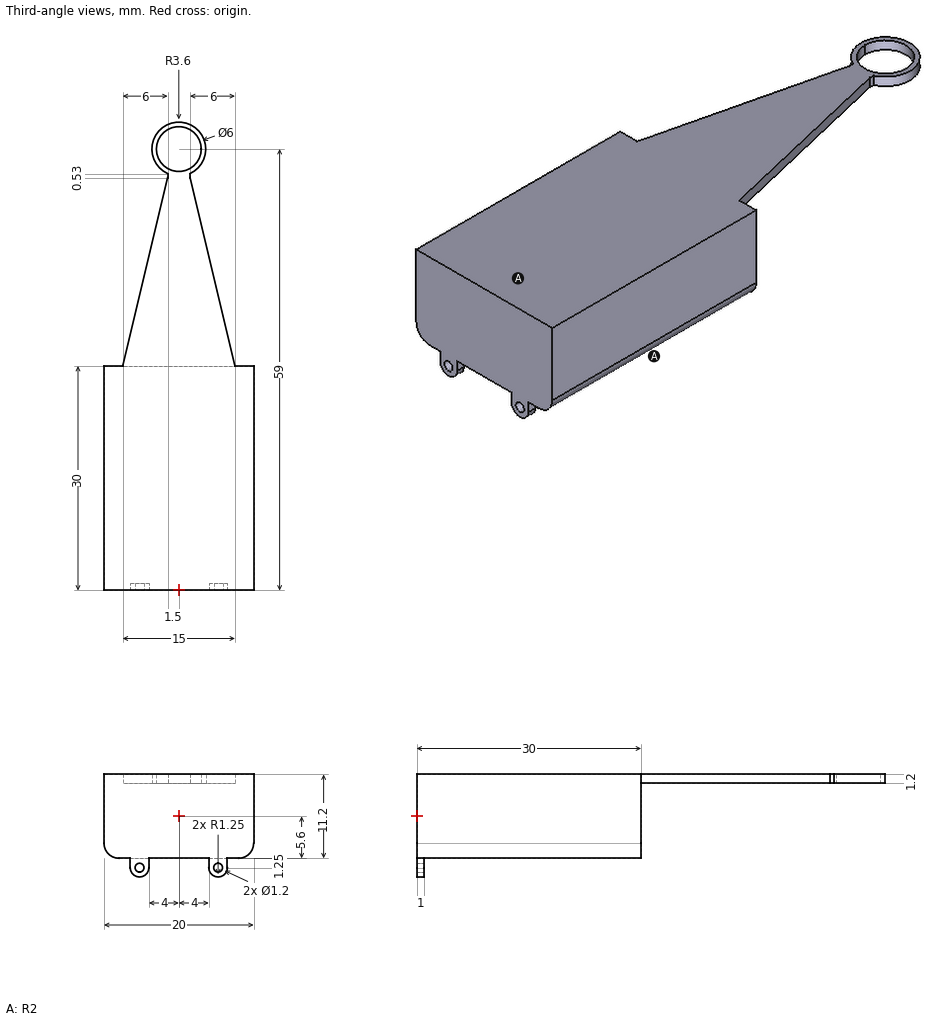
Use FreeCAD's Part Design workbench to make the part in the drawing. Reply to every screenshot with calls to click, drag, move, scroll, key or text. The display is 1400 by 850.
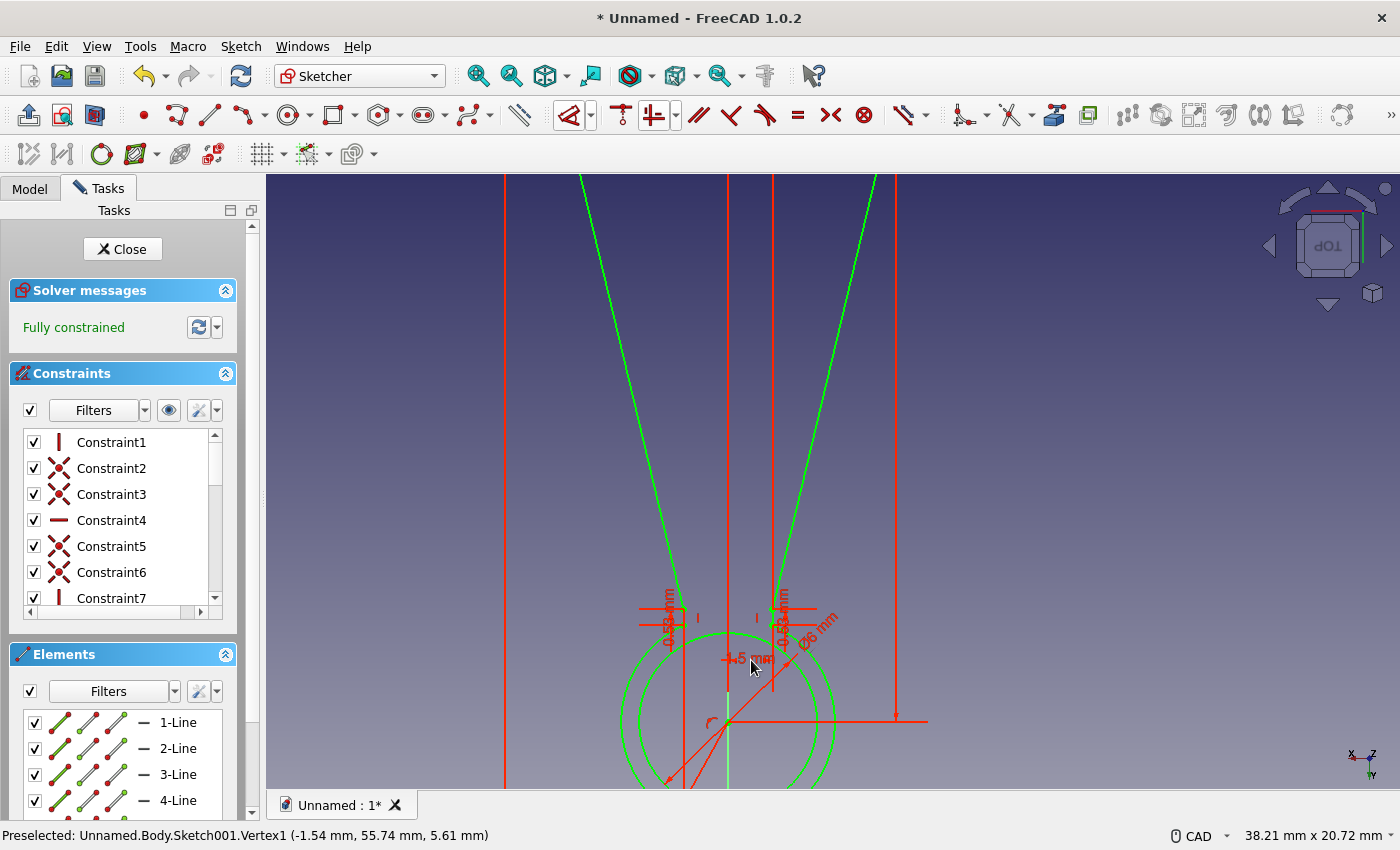
click(123, 249)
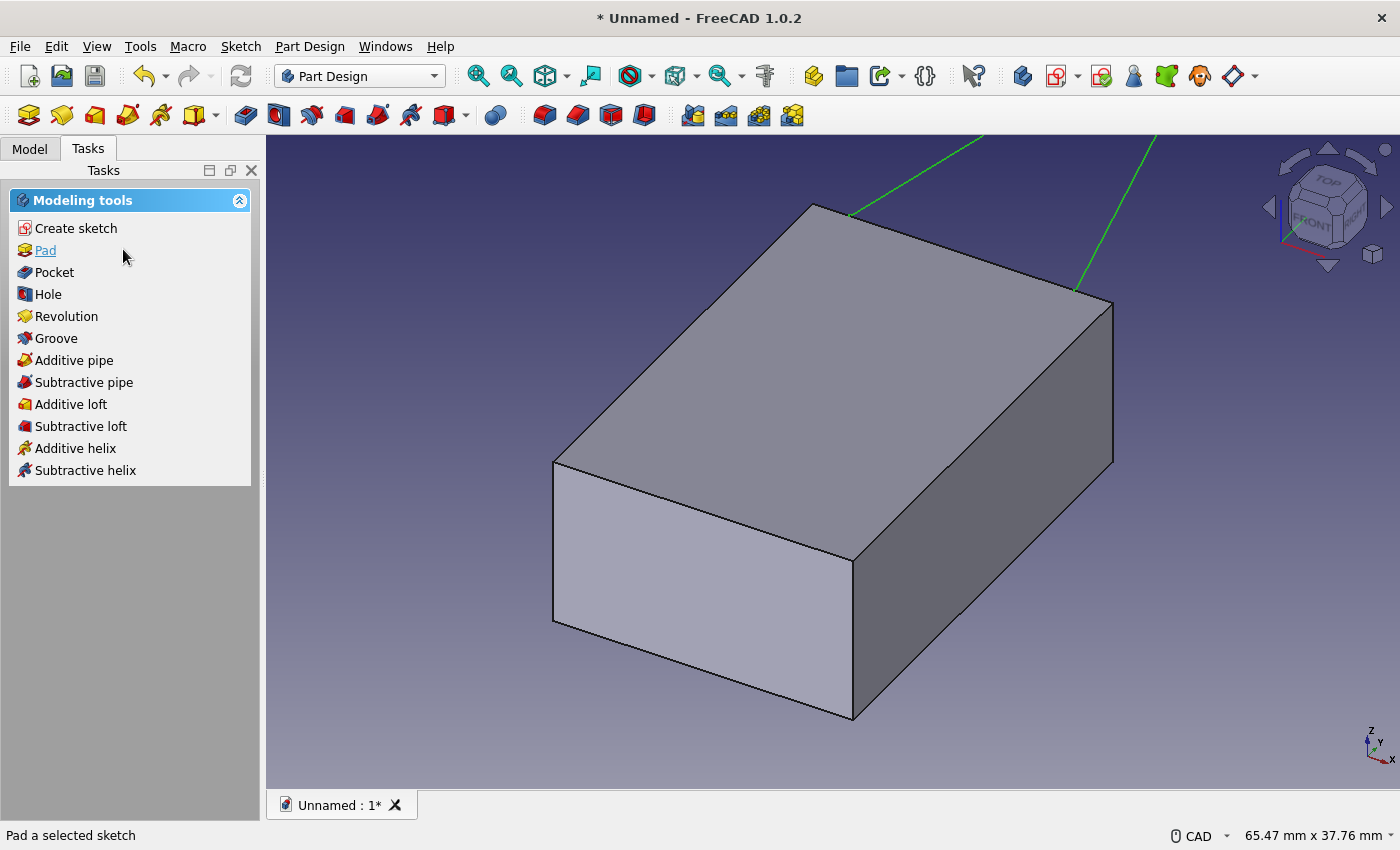
click(29, 116)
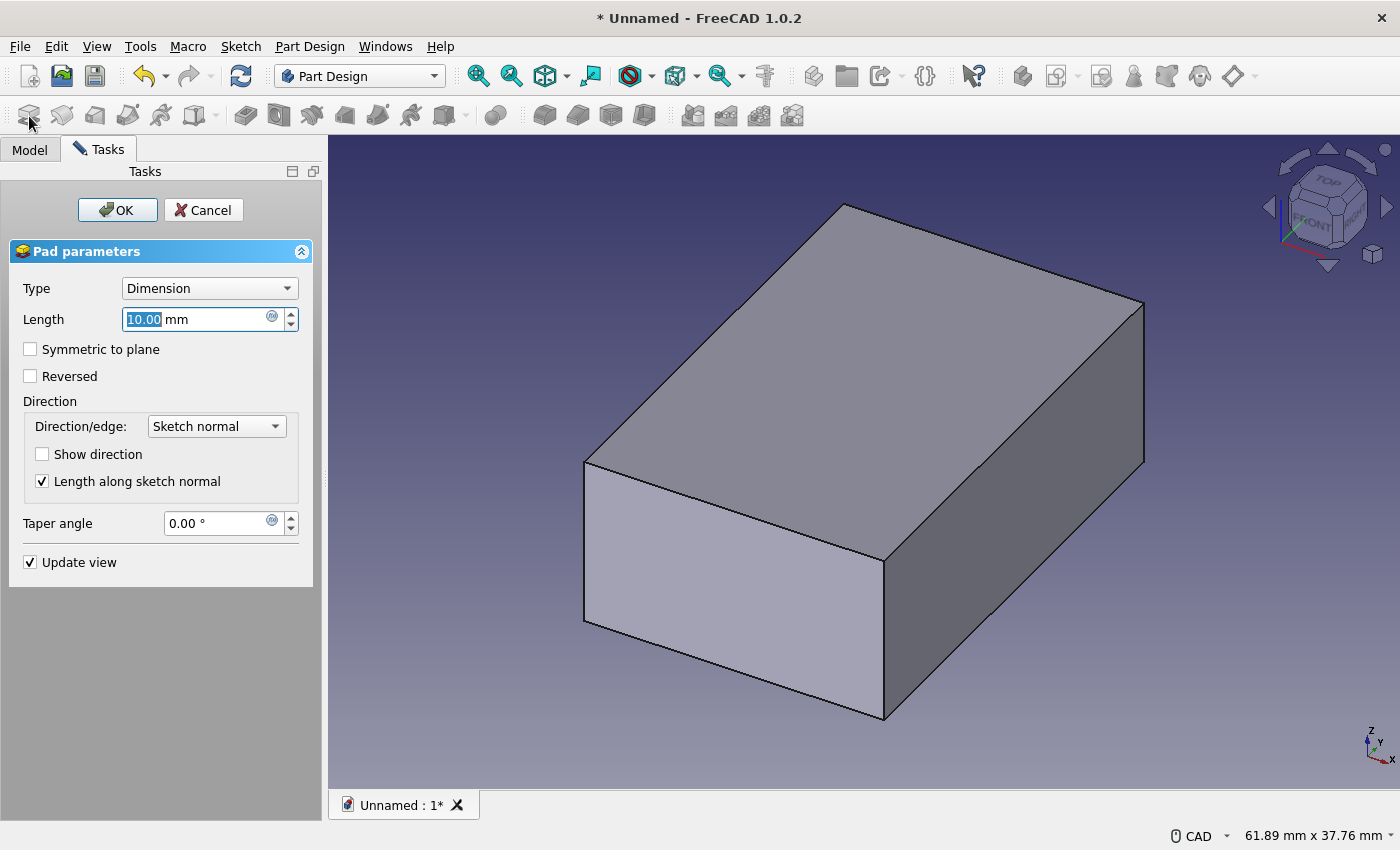
text(1.2)
key(Tab)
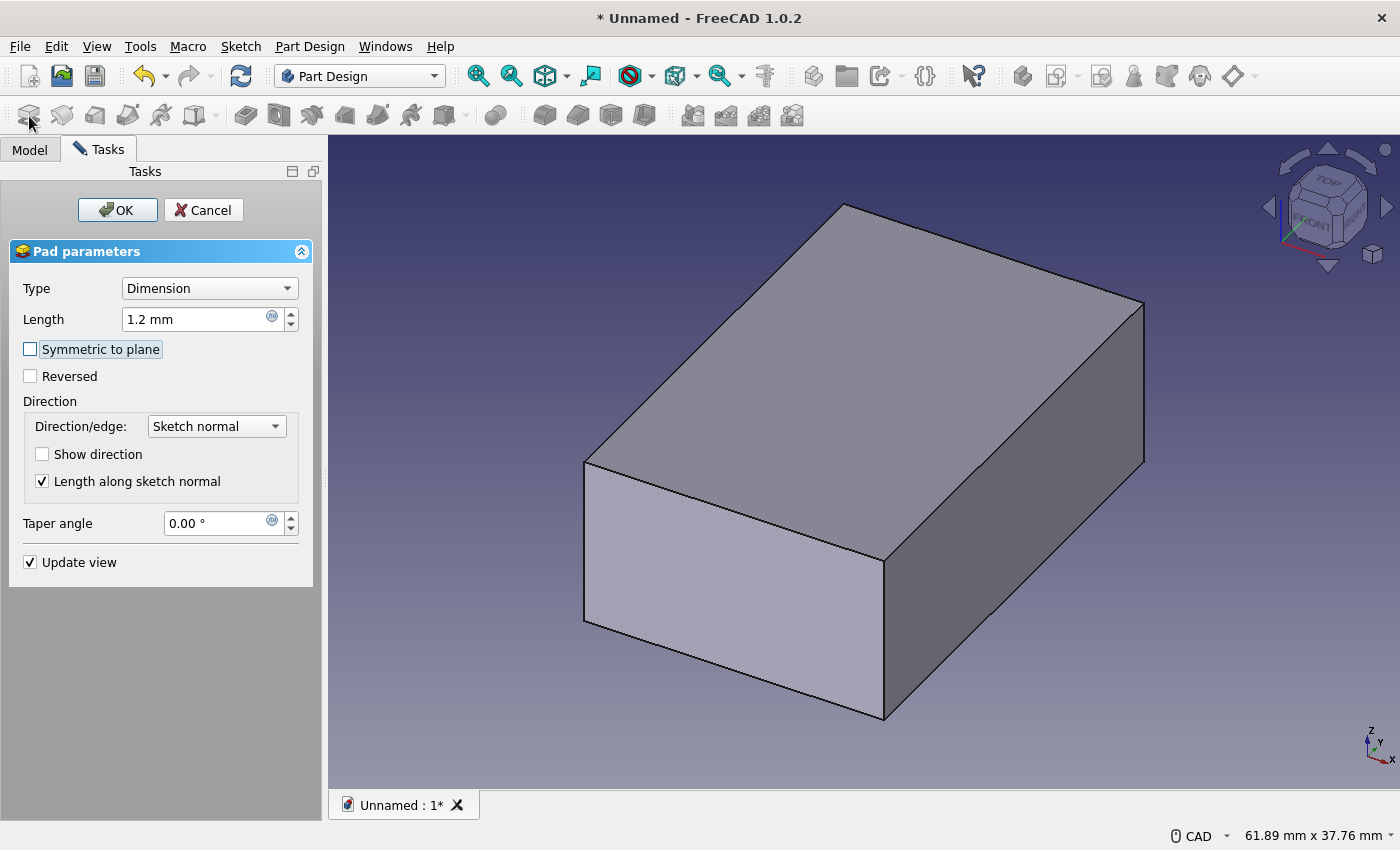
click(31, 376)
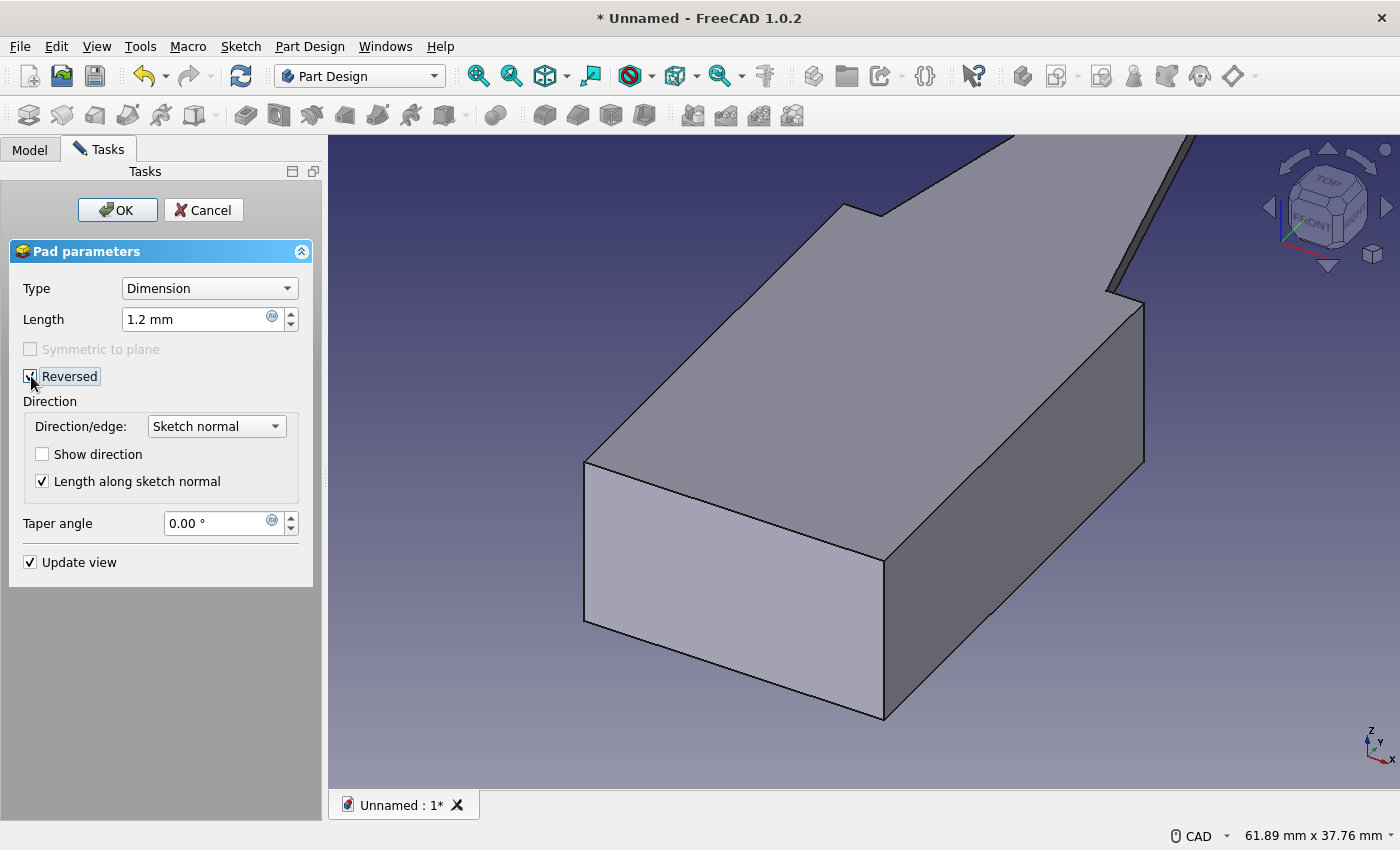
click(118, 210)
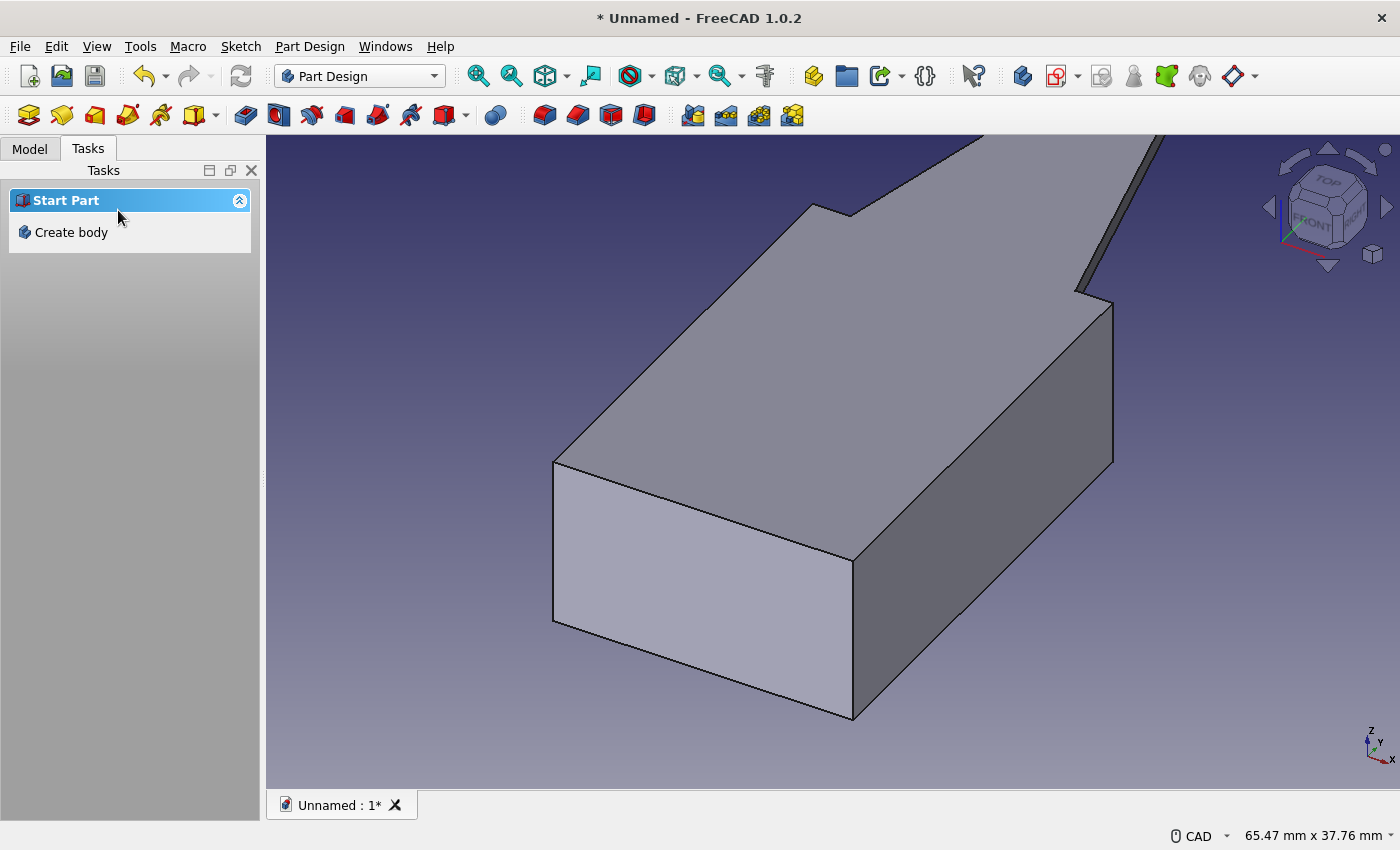
key(v)
key(f)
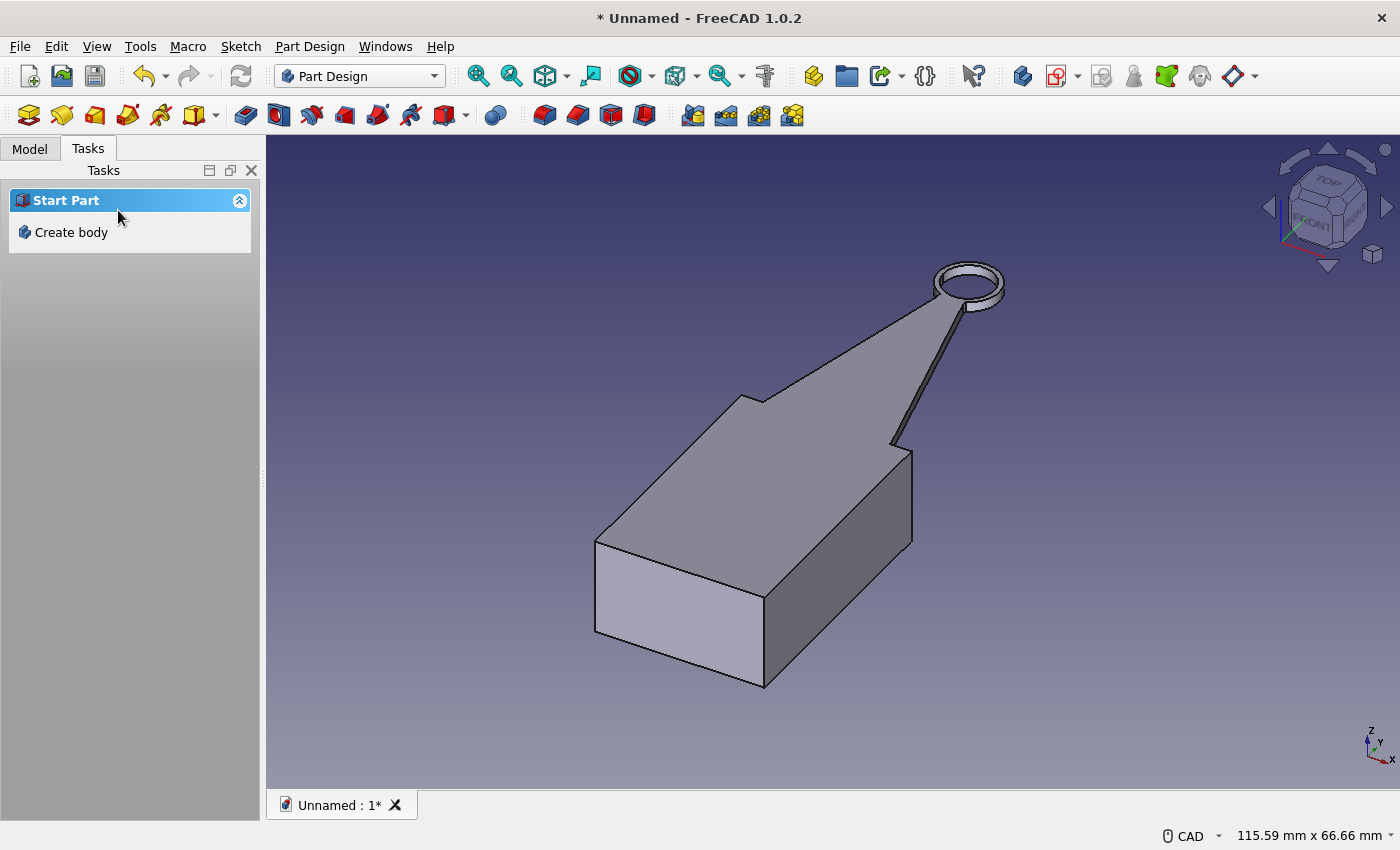
key(0)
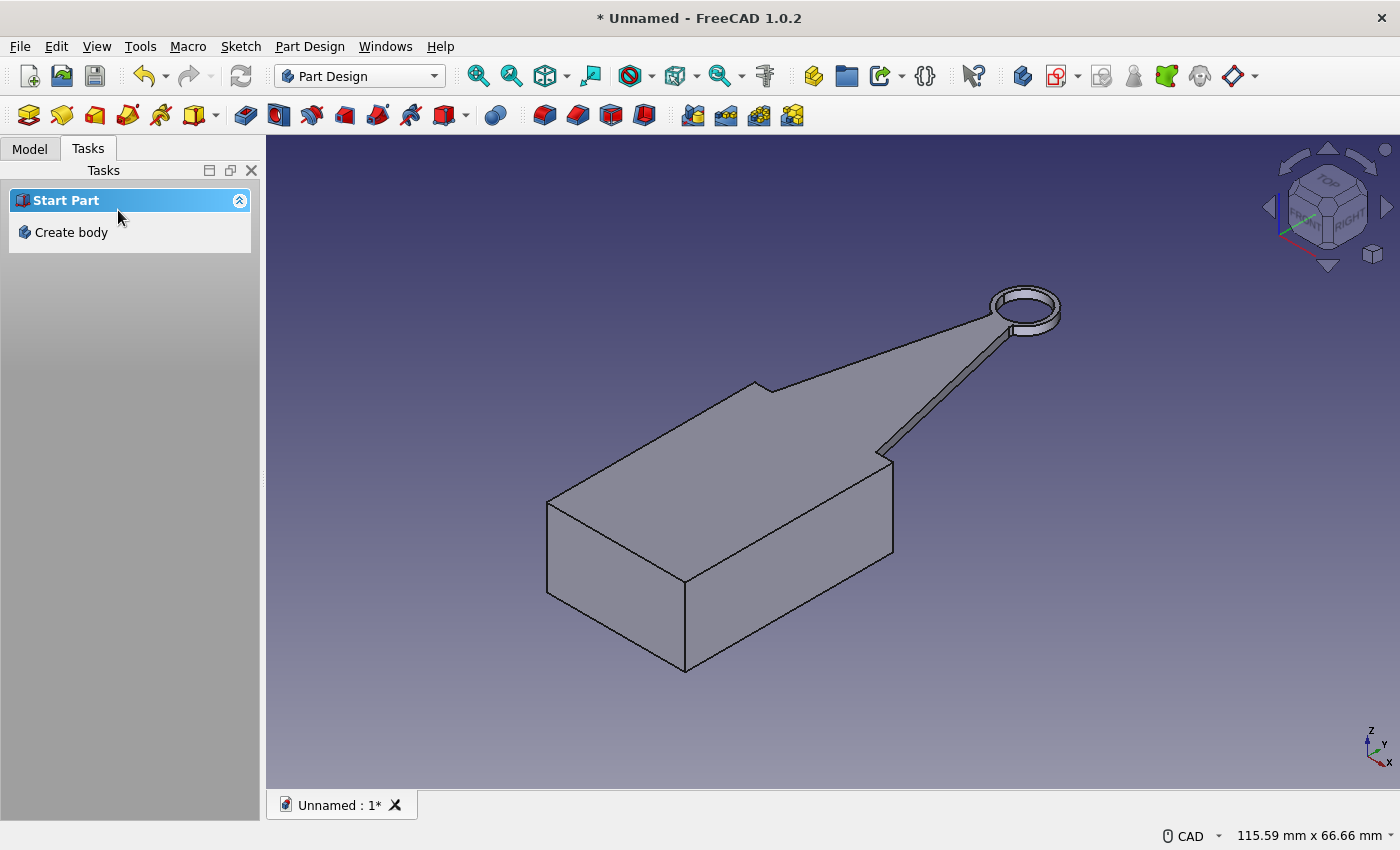
key(2)